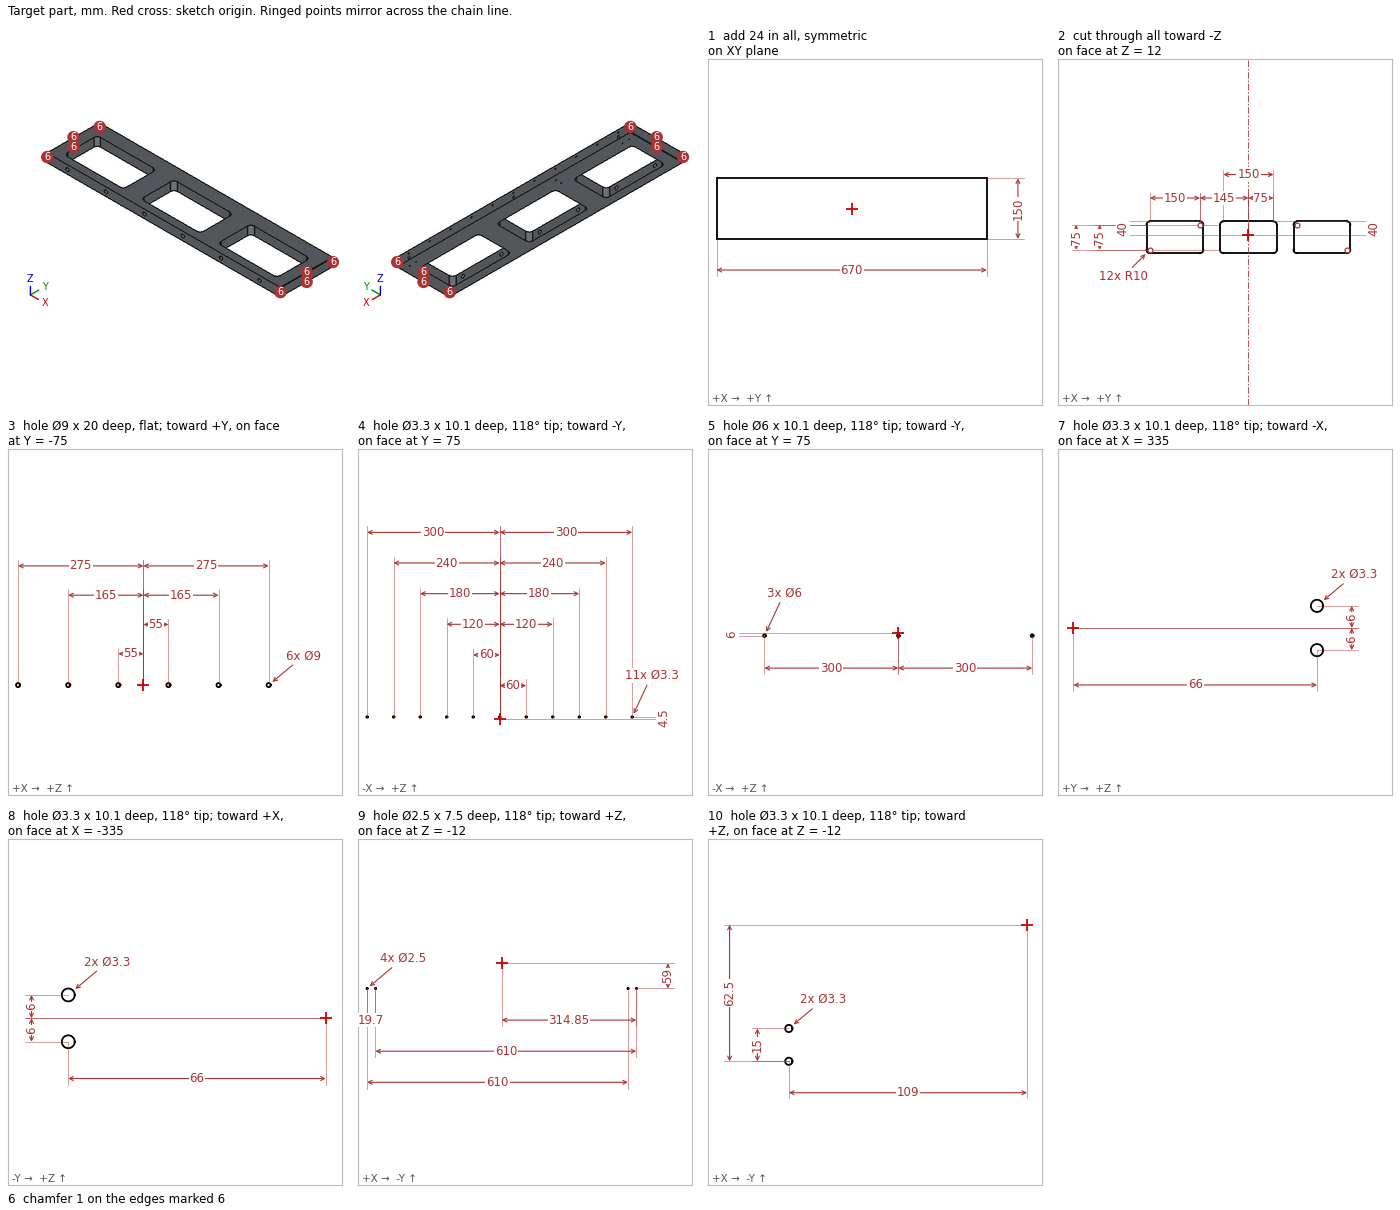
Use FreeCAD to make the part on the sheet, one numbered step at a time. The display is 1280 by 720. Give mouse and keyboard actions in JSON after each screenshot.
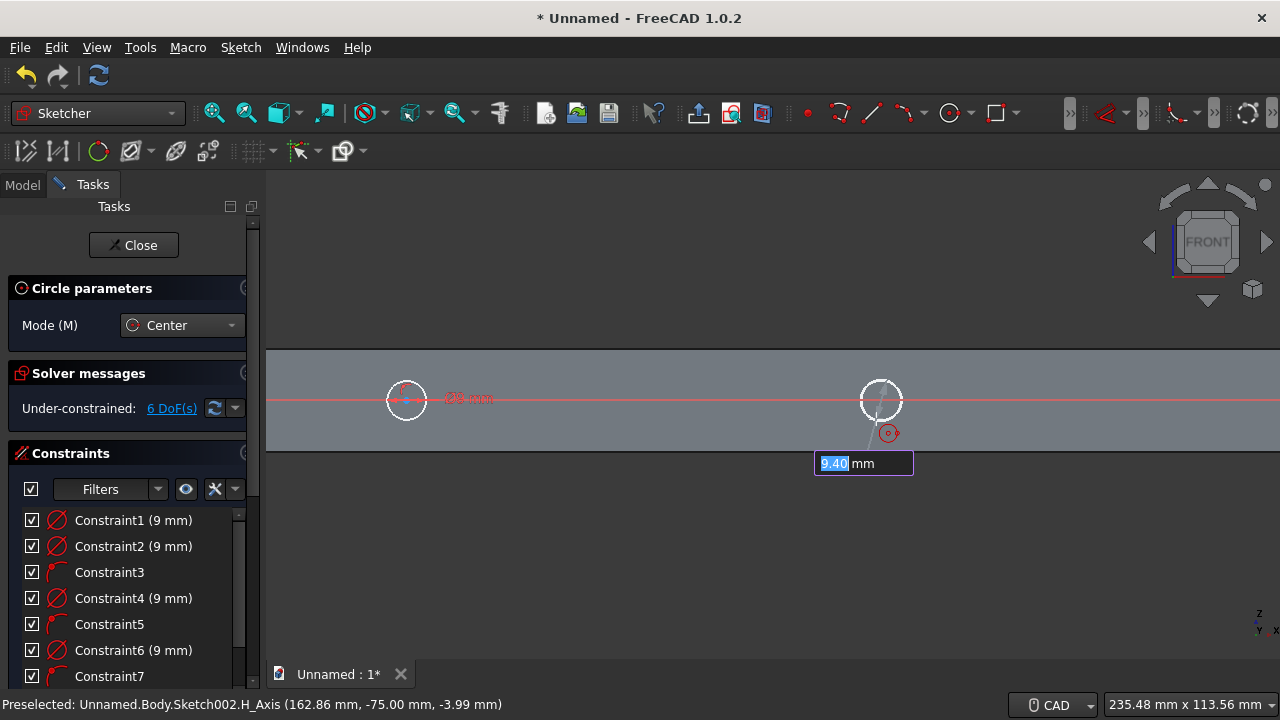
{"action": "type", "text": "9"}
{"action": "key", "text": "Return"}
{"action": "key", "text": "Escape"}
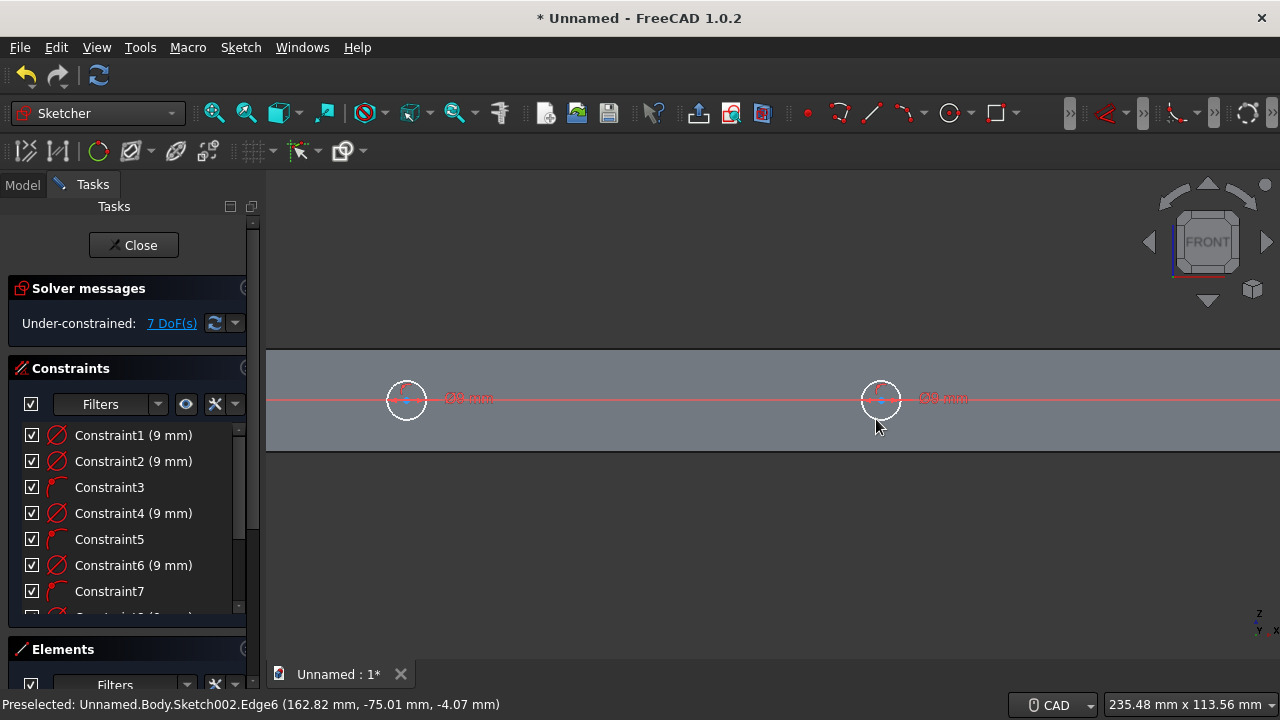
{"action": "scroll", "coordinate": [879, 419], "scroll_direction": "down", "scroll_amount": 7}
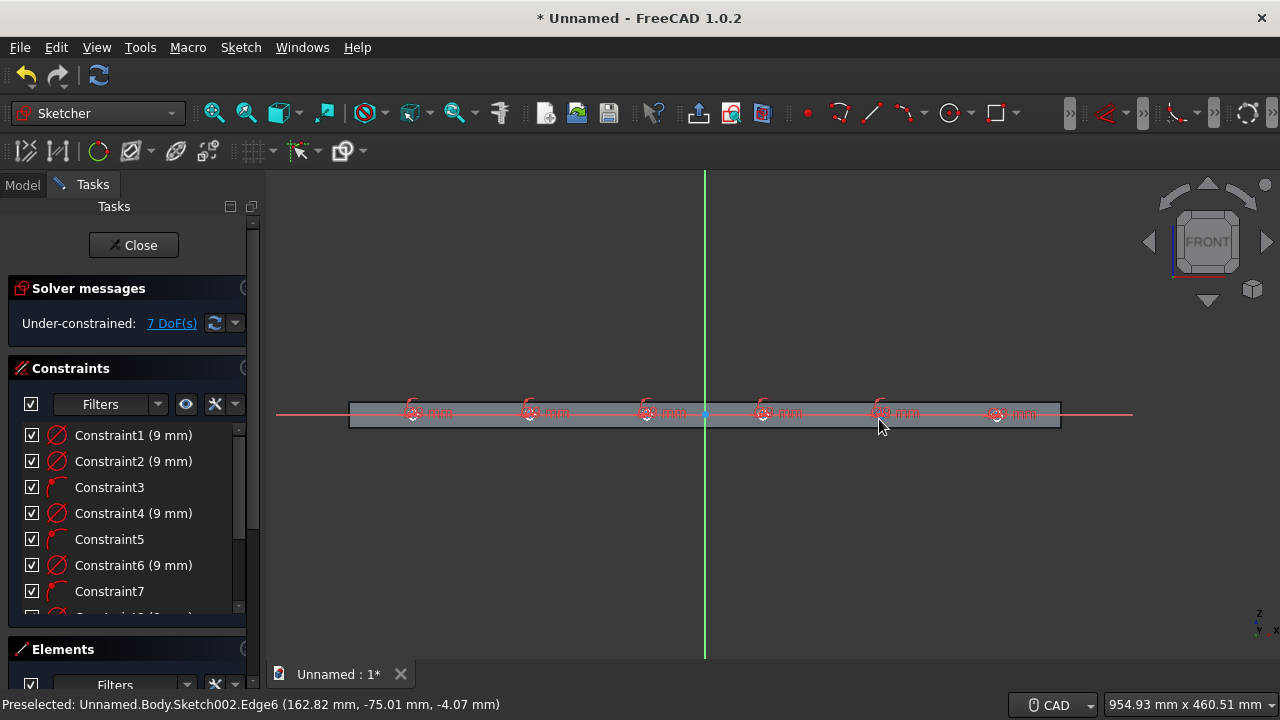
{"action": "left_click", "coordinate": [997, 416]}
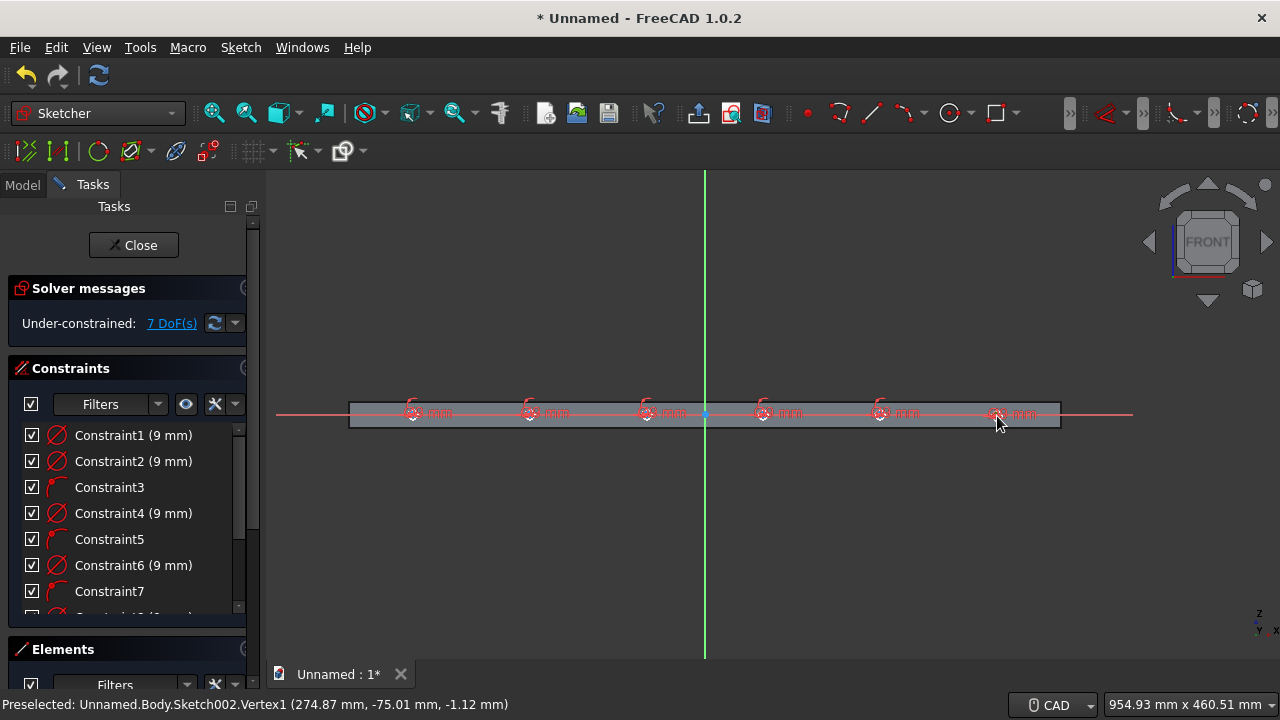
{"action": "left_click", "coordinate": [353, 415]}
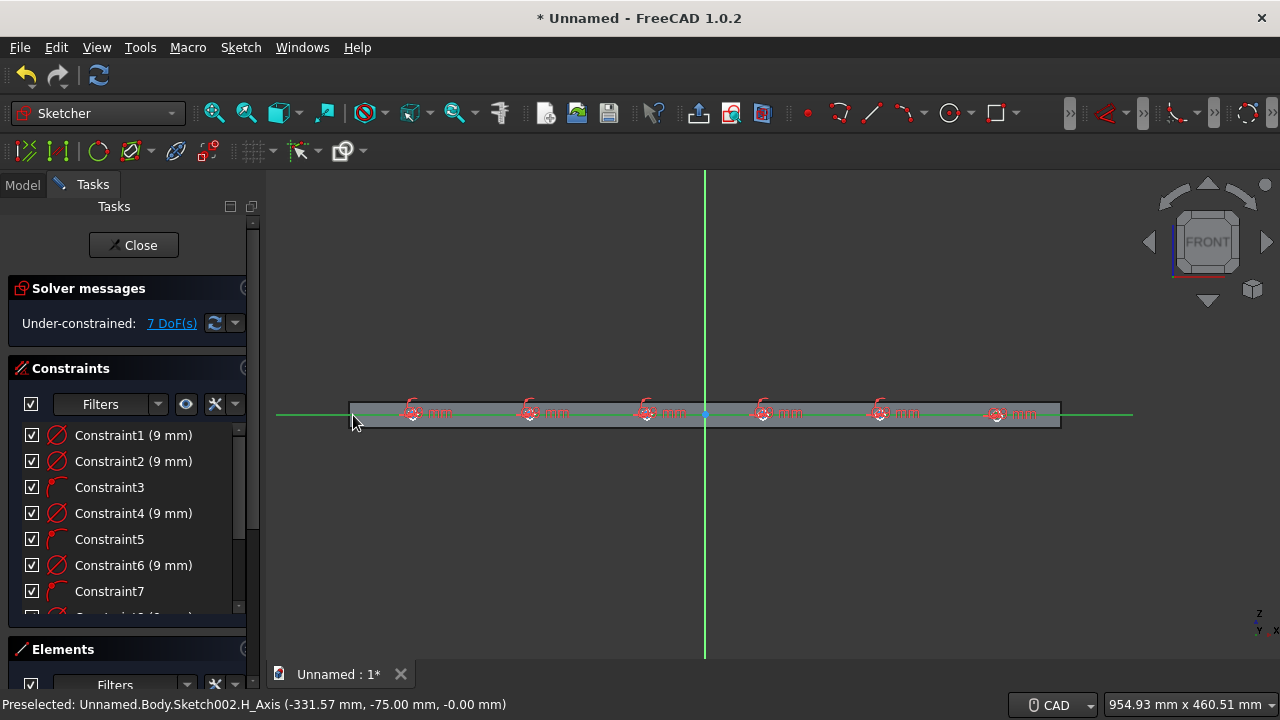
{"action": "key", "text": "c"}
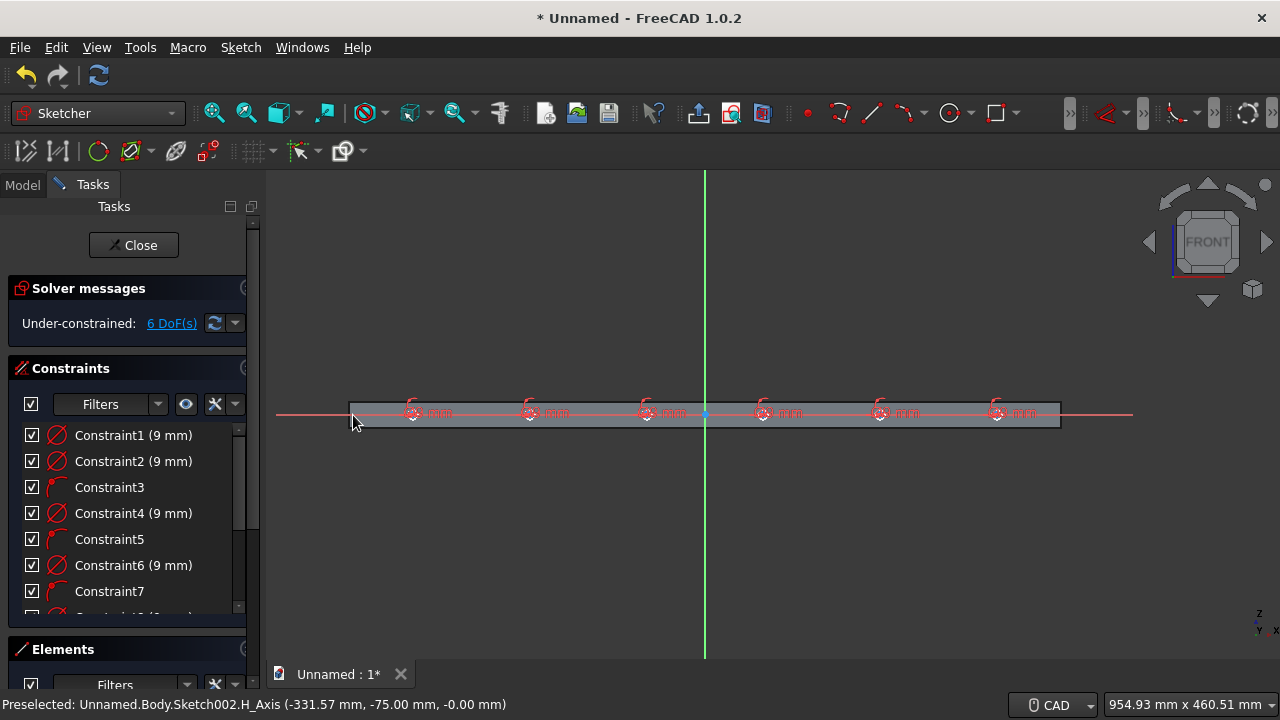
{"action": "left_click", "coordinate": [1106, 114]}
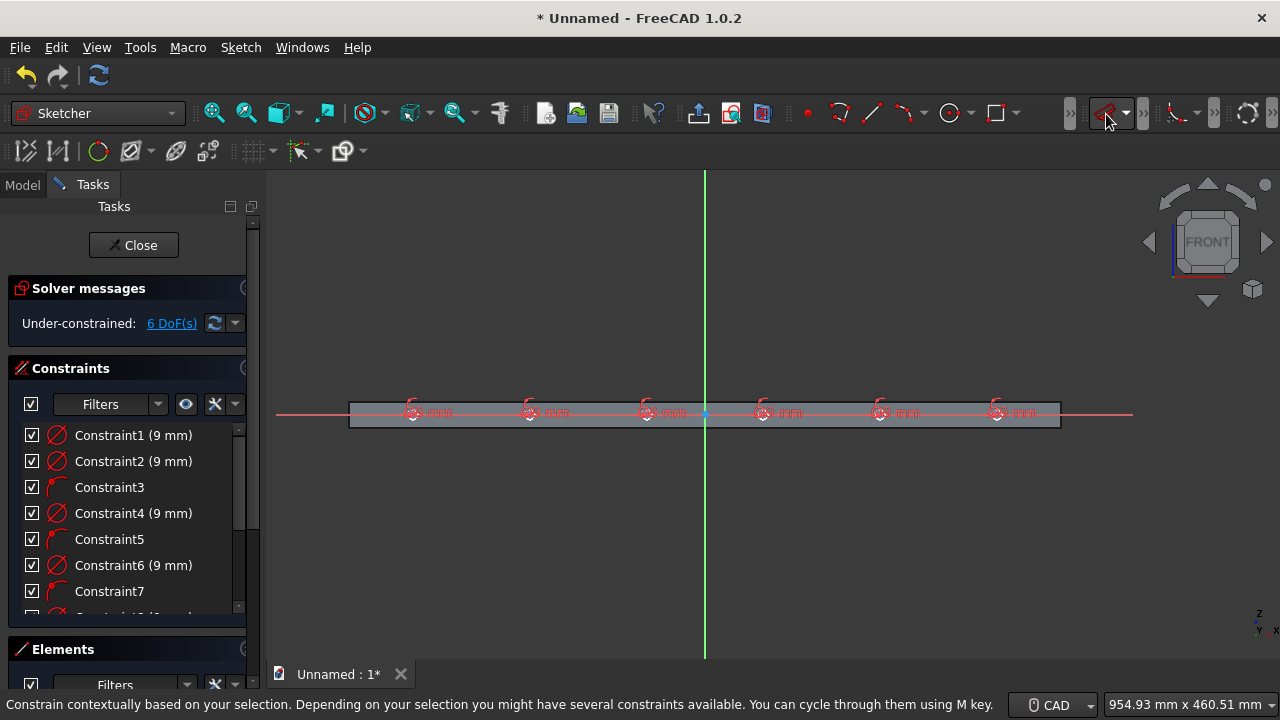
{"action": "left_click", "coordinate": [647, 415]}
{"action": "left_click", "coordinate": [676, 449]}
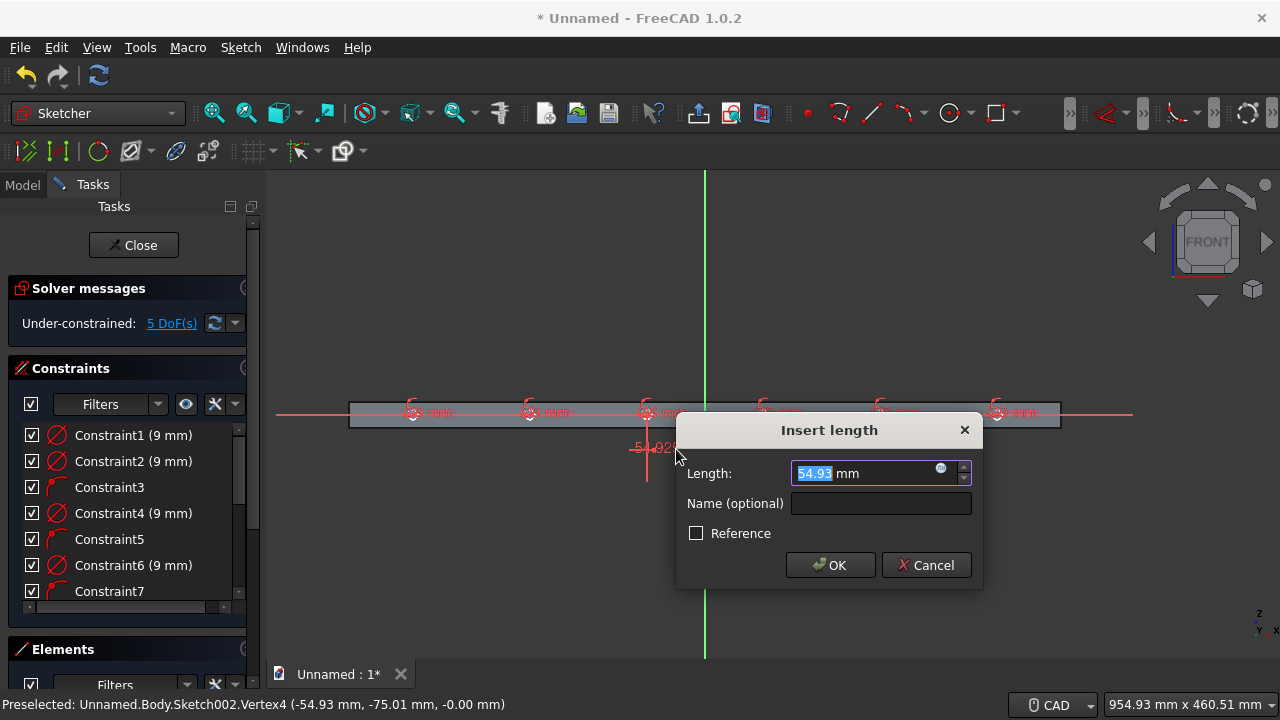
{"action": "type", "text": "55"}
{"action": "key", "text": "Return"}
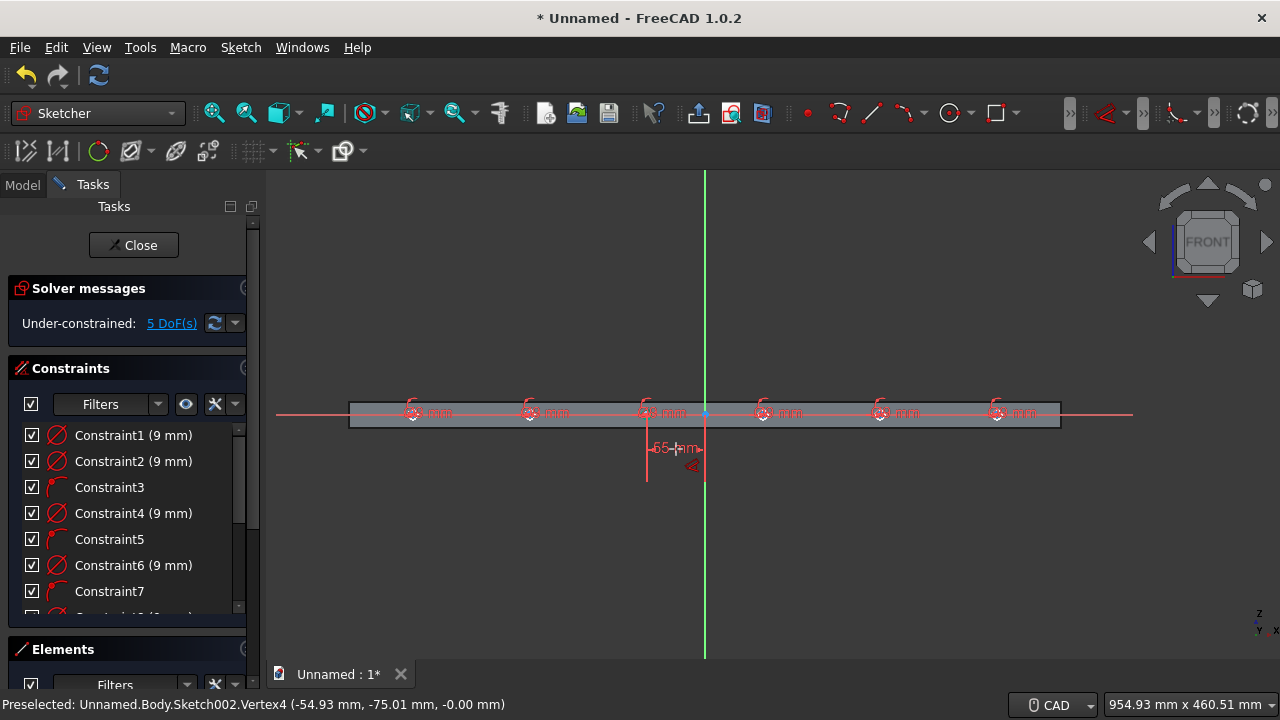
{"action": "left_click", "coordinate": [763, 415]}
{"action": "left_click", "coordinate": [747, 449]}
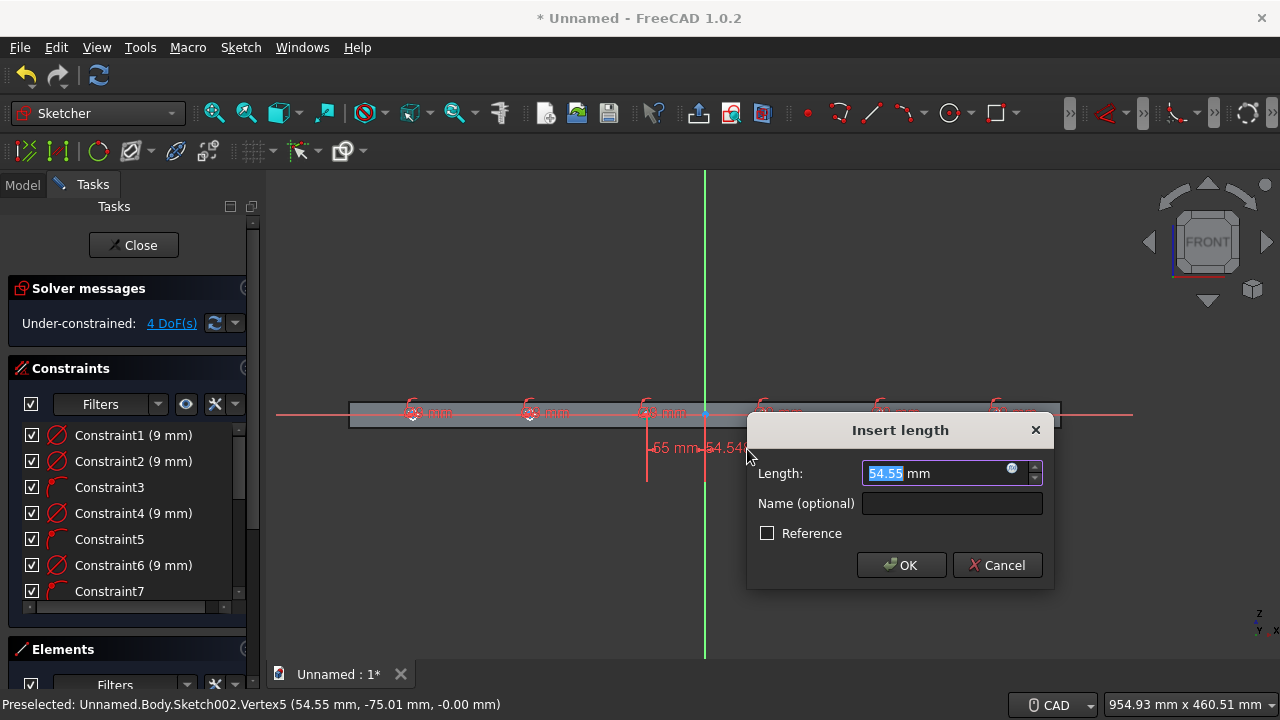
{"action": "type", "text": "55"}
{"action": "key", "text": "Return"}